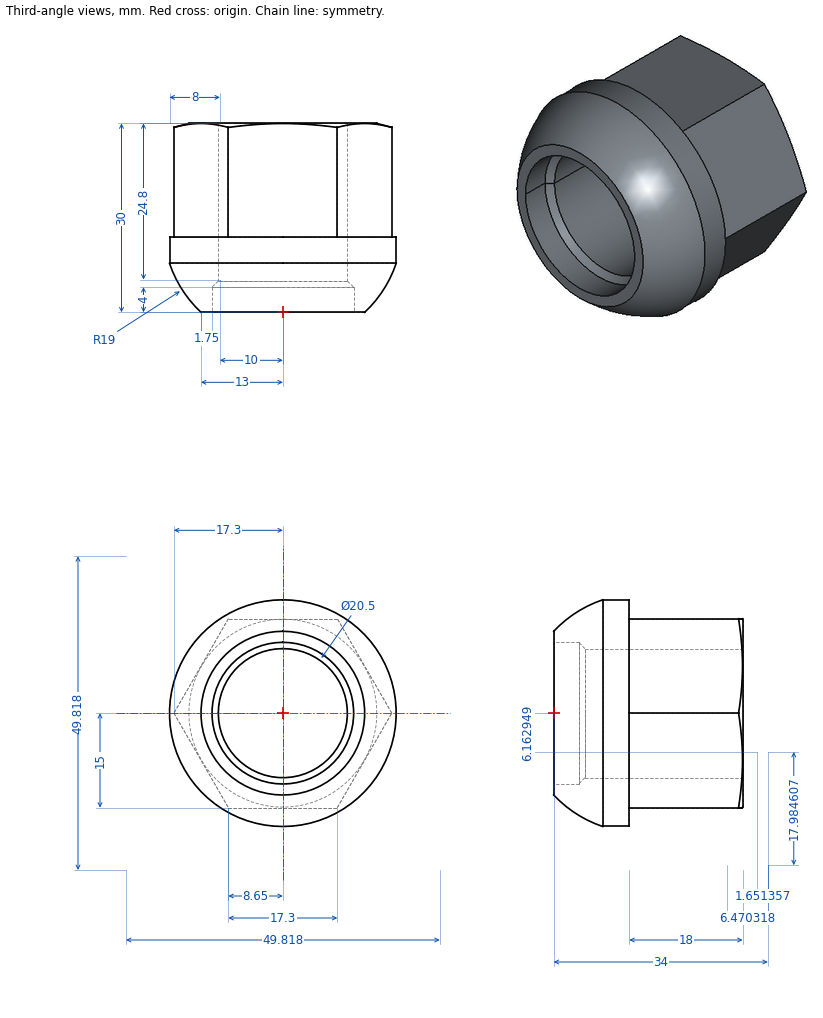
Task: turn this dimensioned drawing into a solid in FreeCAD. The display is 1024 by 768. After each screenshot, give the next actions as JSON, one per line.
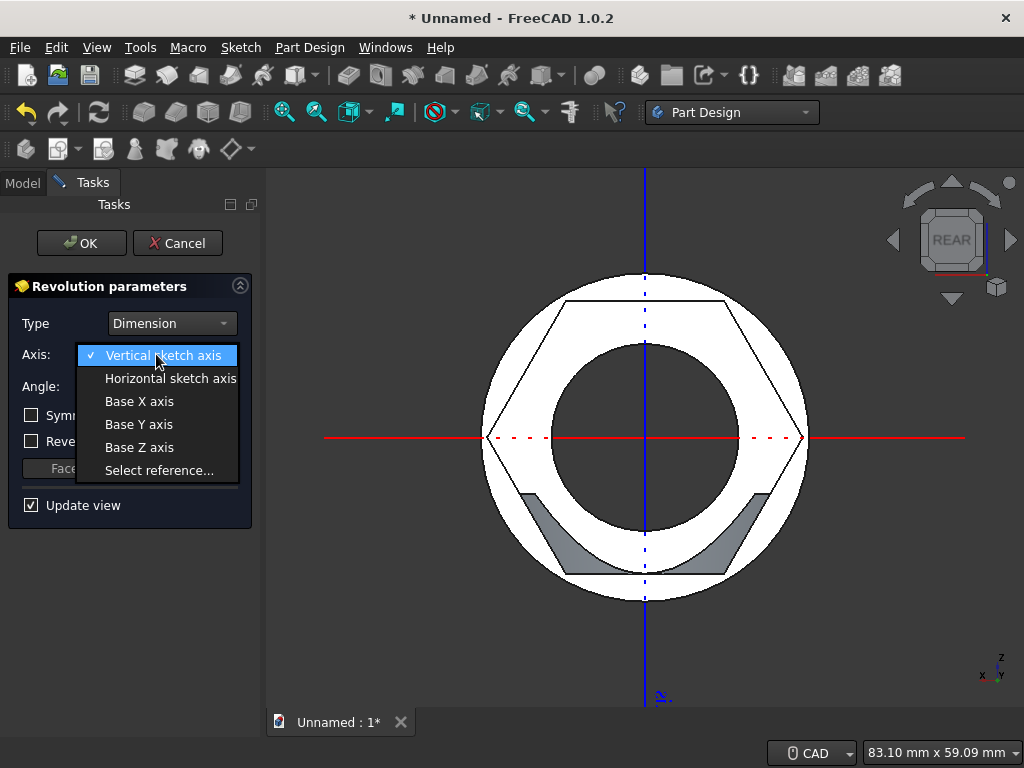
{"action": "left_click", "coordinate": [156, 378]}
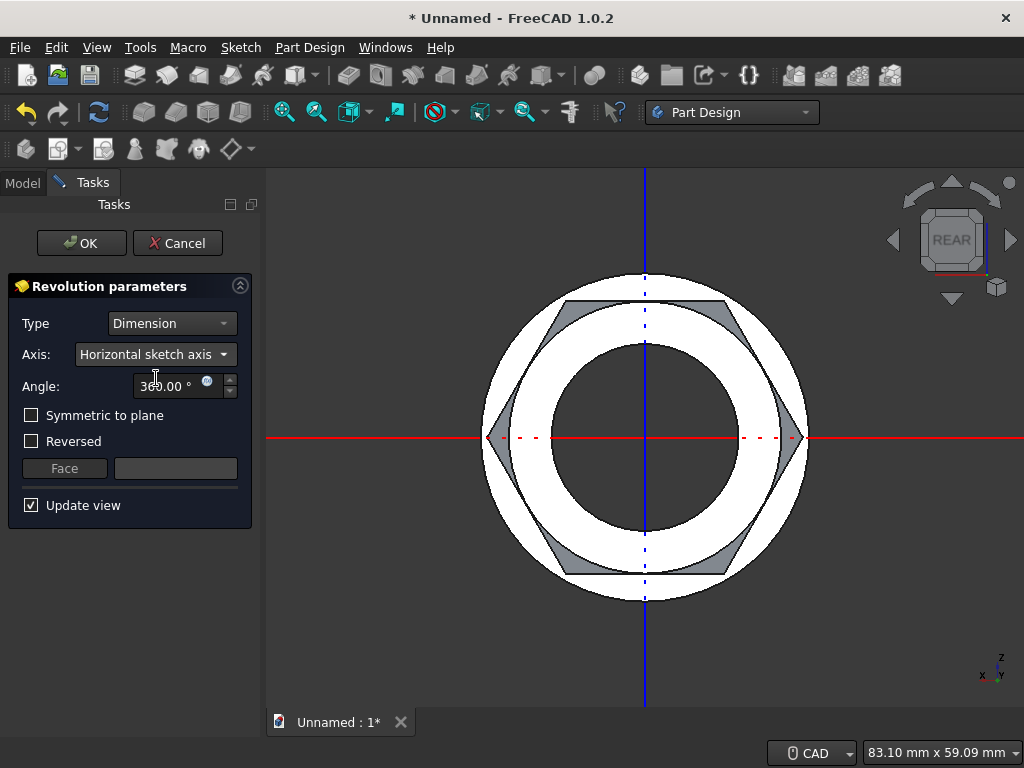
{"action": "left_click", "coordinate": [82, 243]}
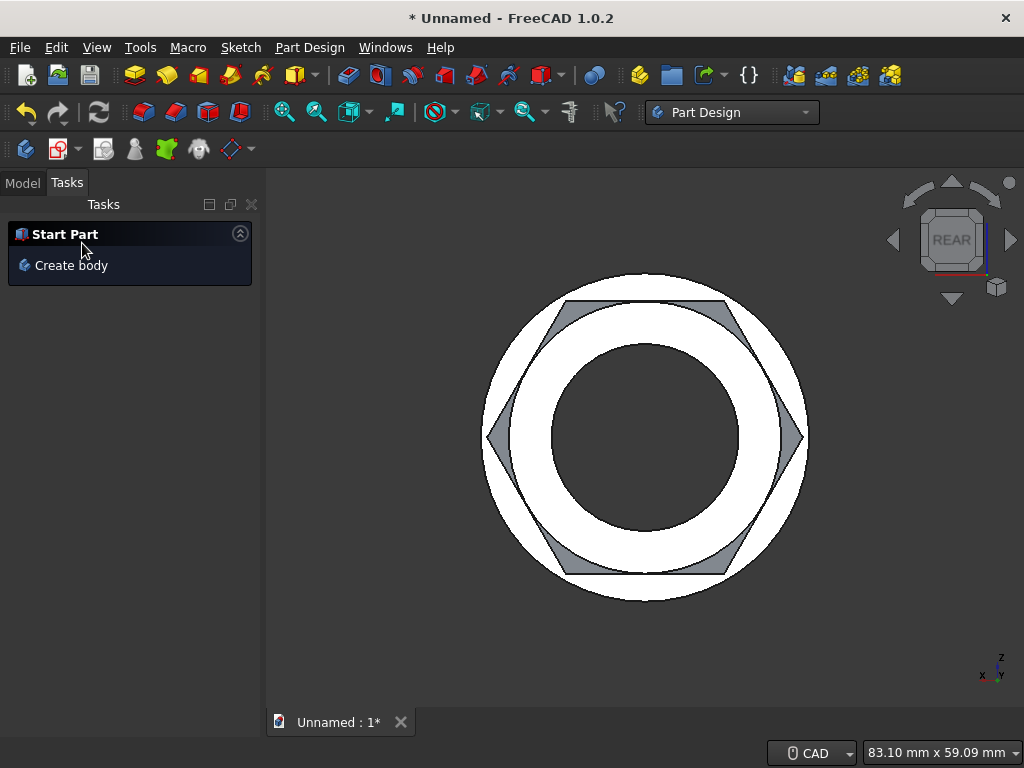
{"action": "key", "text": "0"}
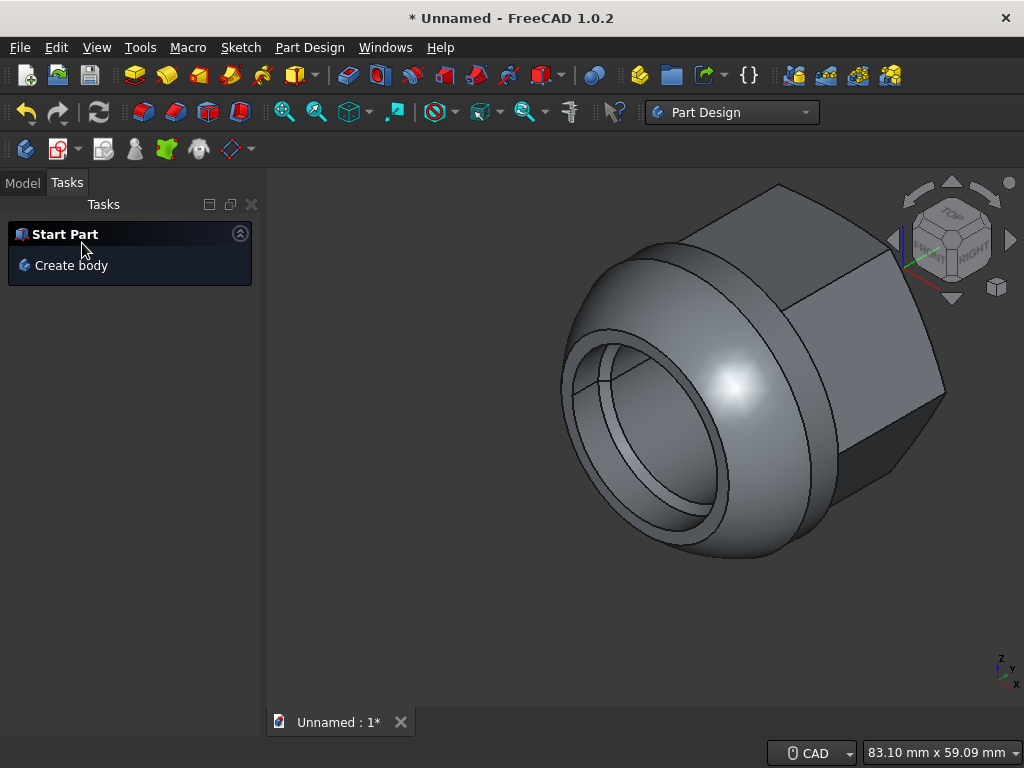
{"action": "left_click", "coordinate": [286, 112]}